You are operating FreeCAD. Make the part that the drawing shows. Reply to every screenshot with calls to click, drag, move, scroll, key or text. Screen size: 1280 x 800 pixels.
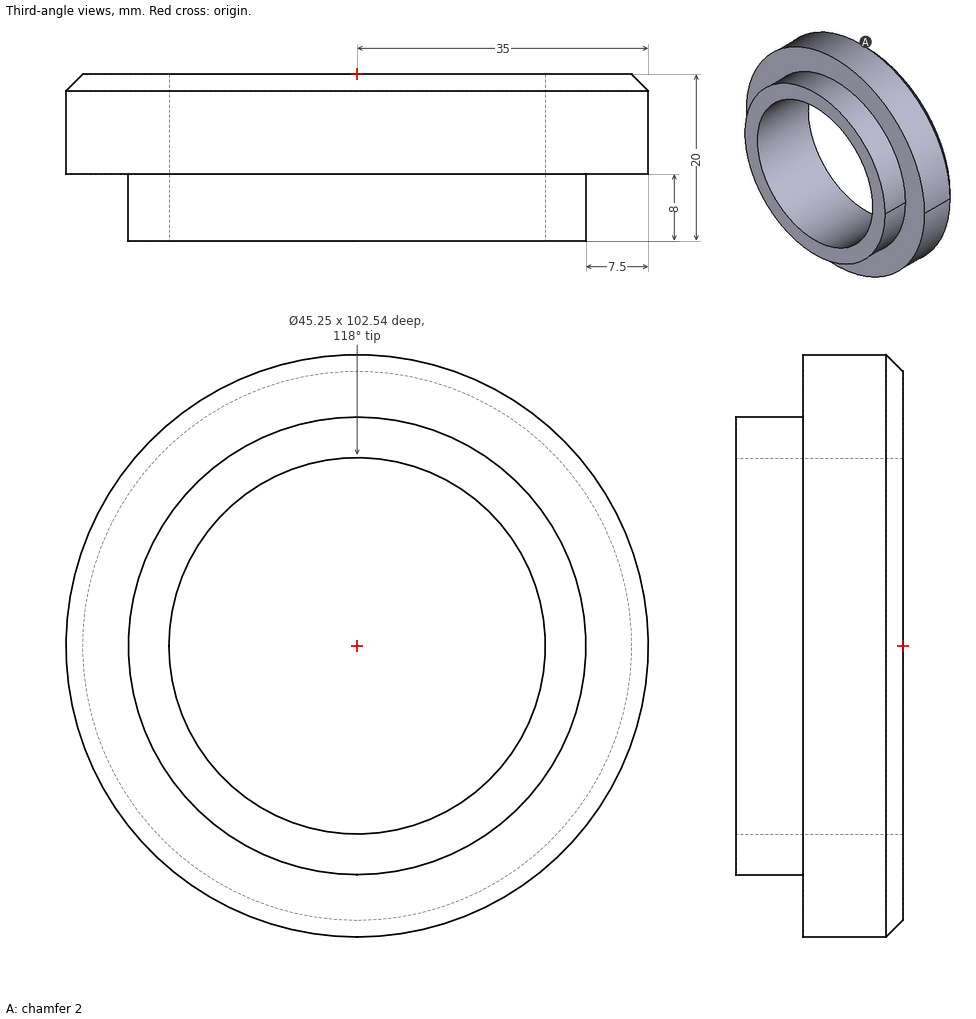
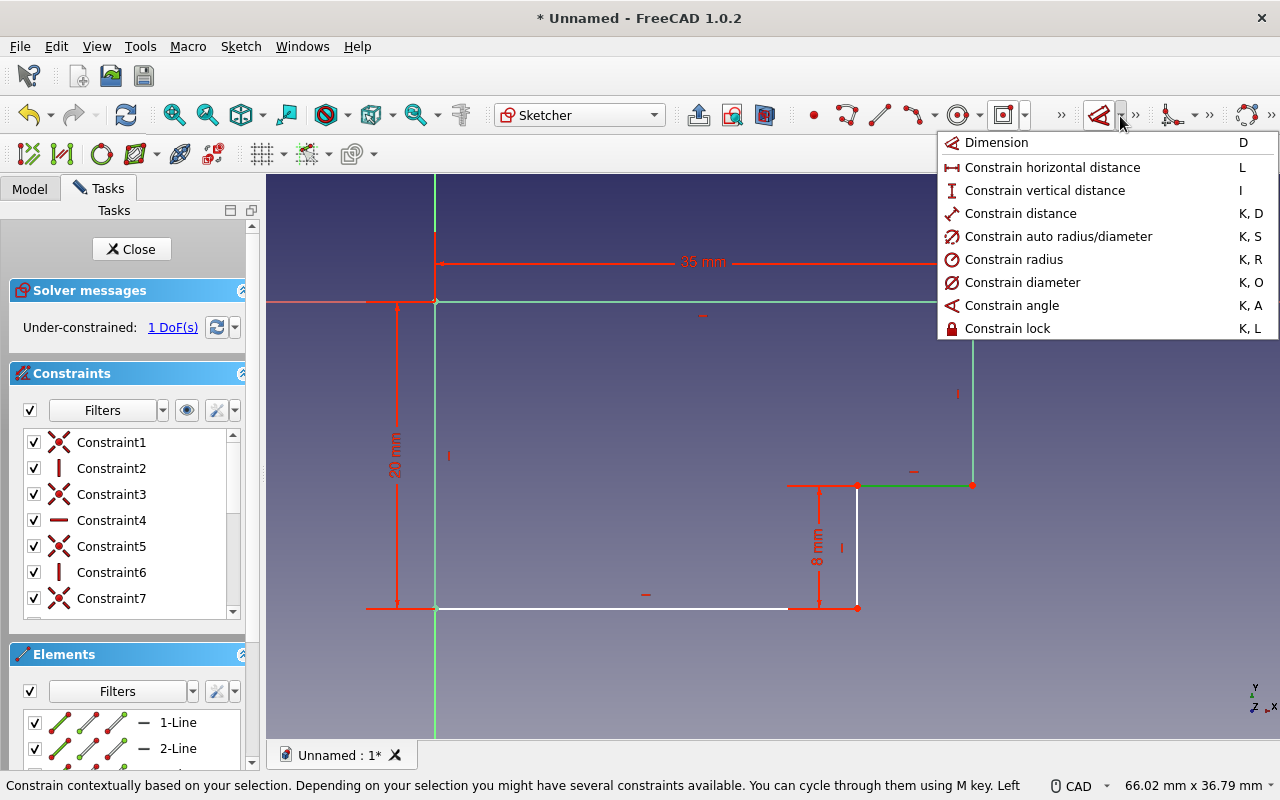
click(1108, 168)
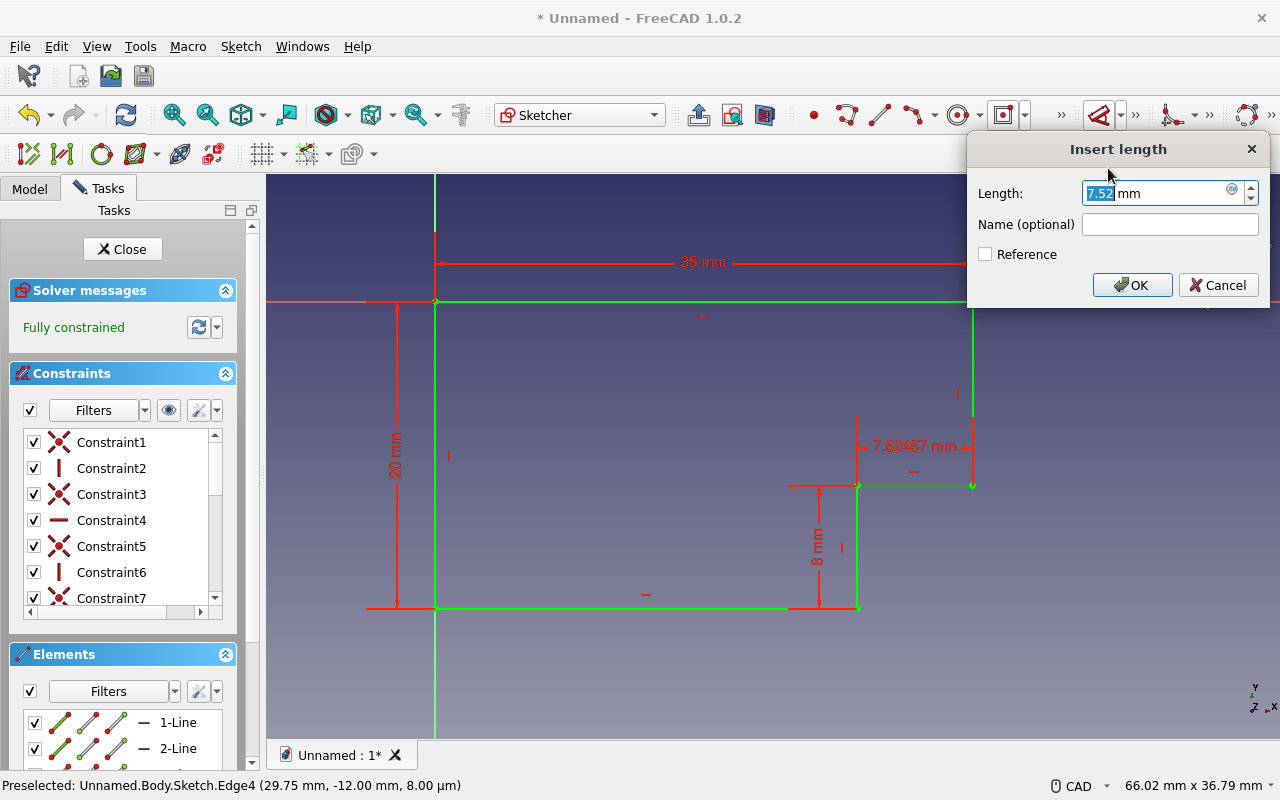
text(7.5)
key(Return)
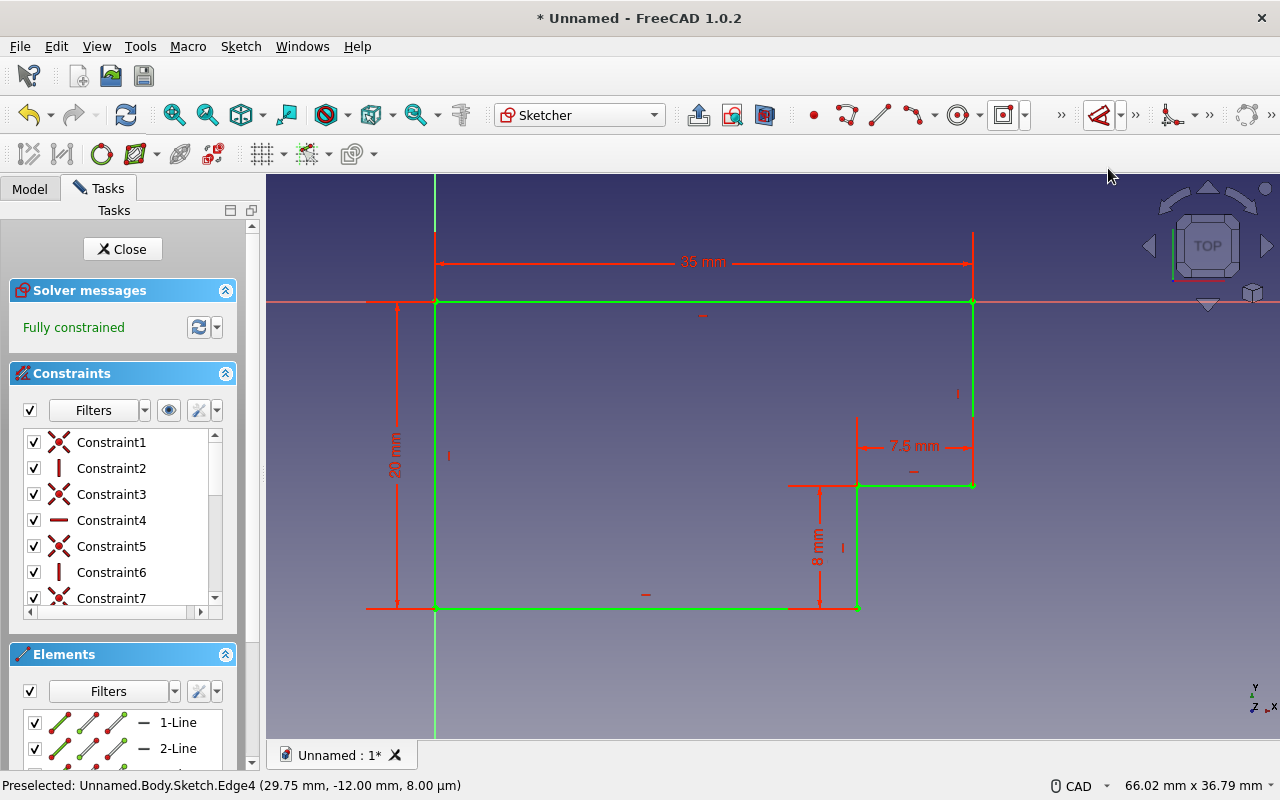
click(123, 249)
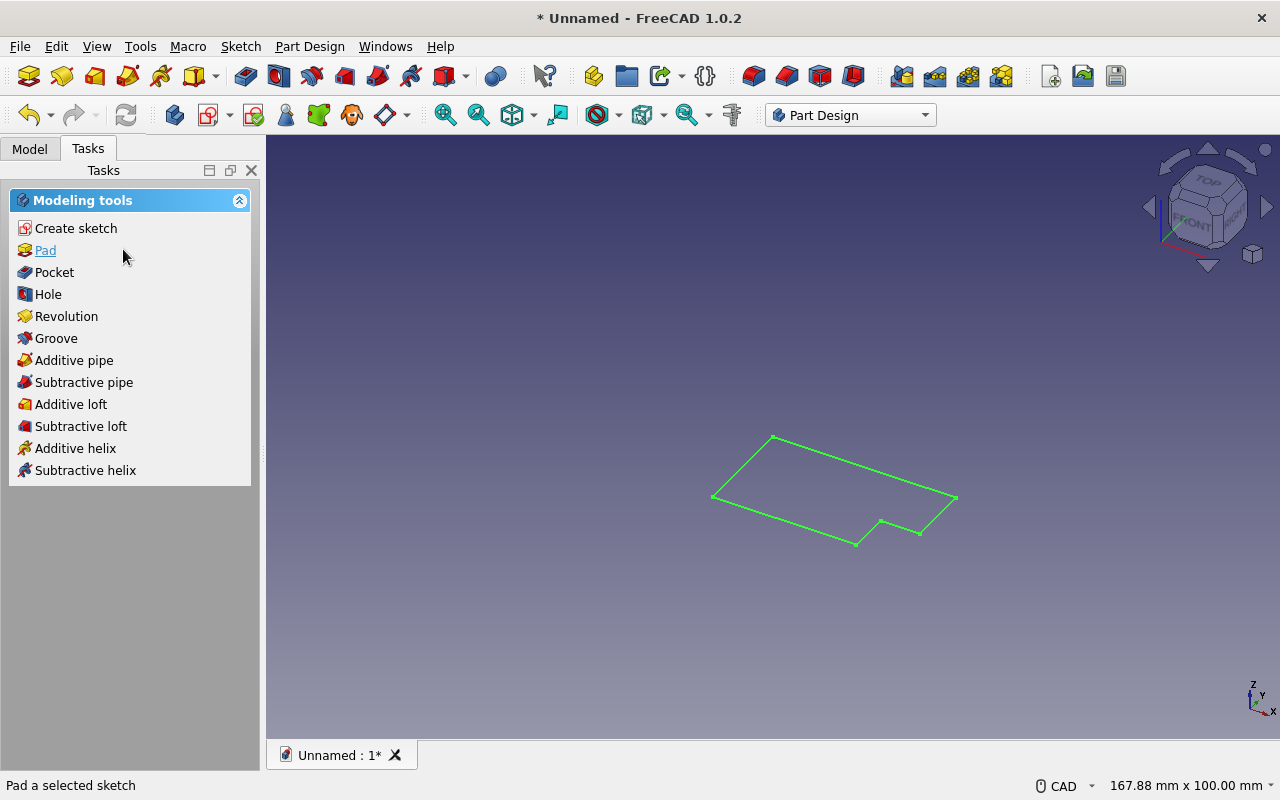
click(62, 76)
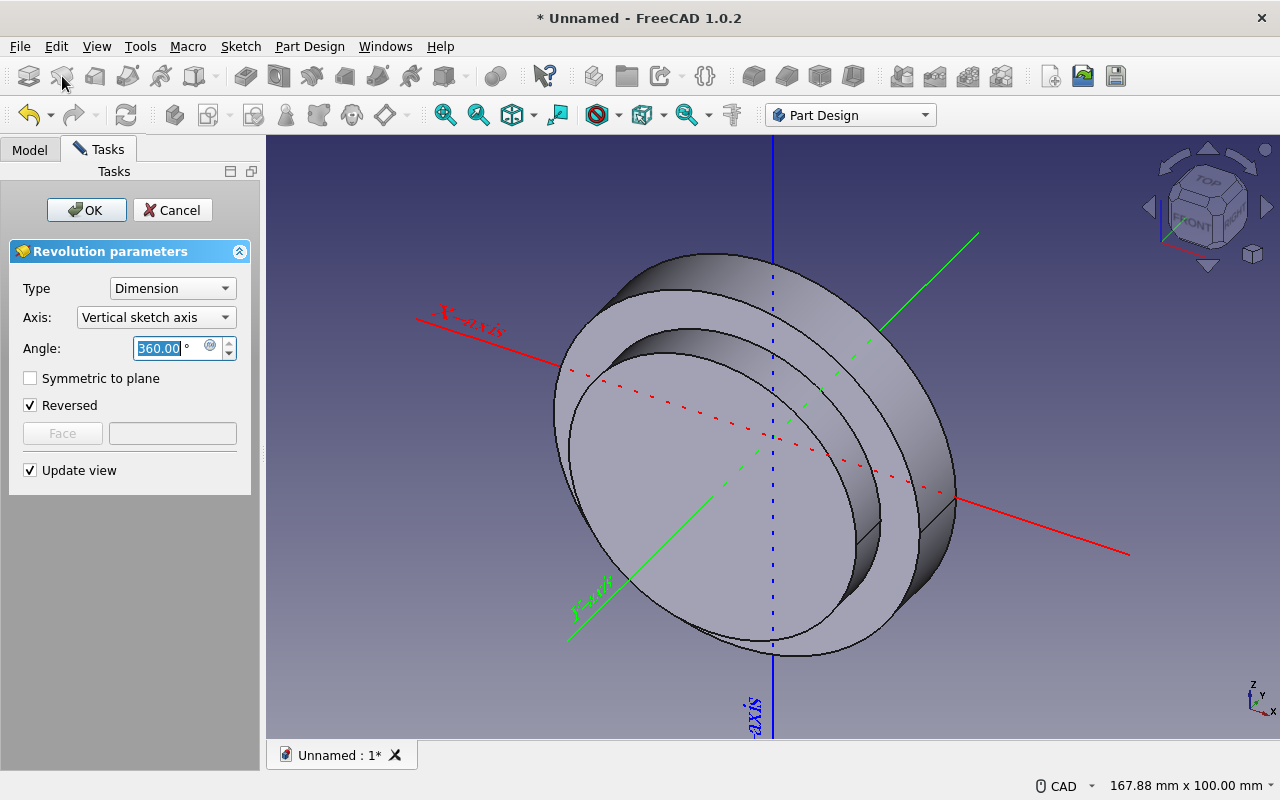
click(87, 210)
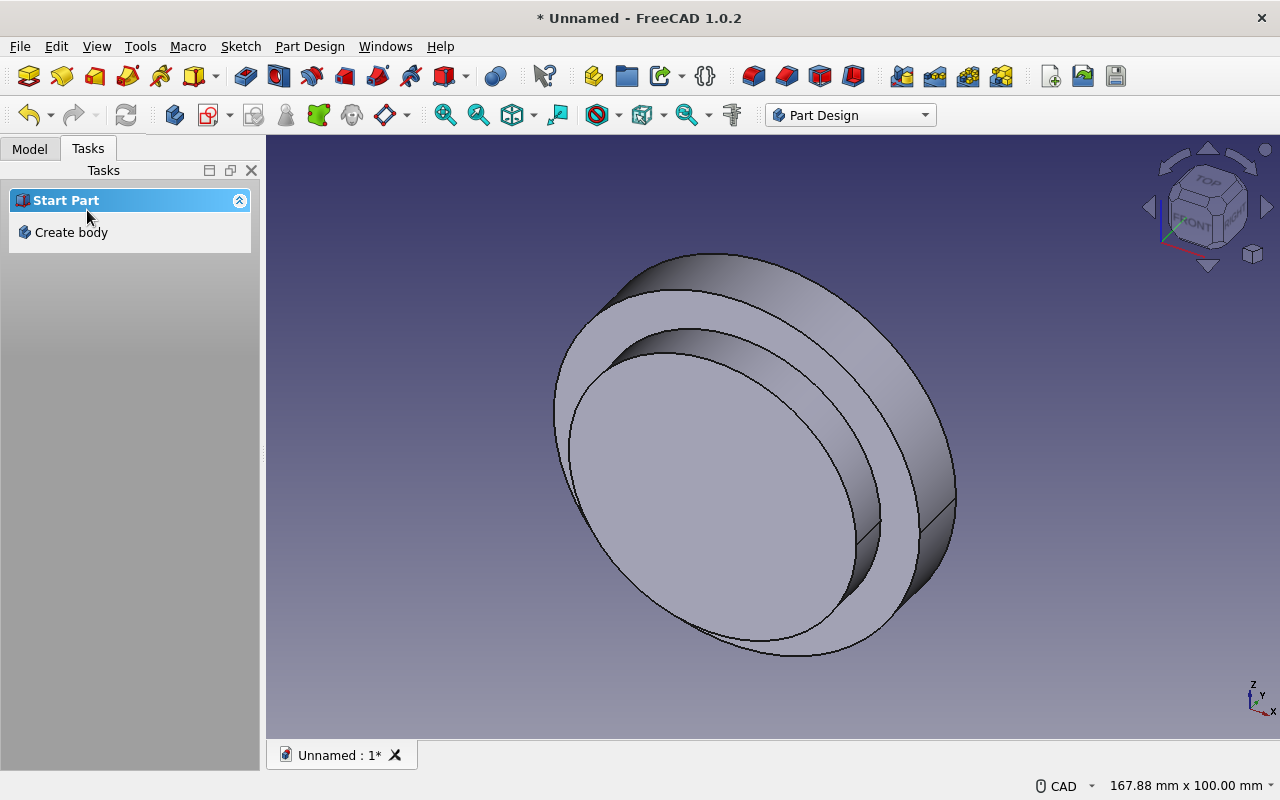
click(208, 116)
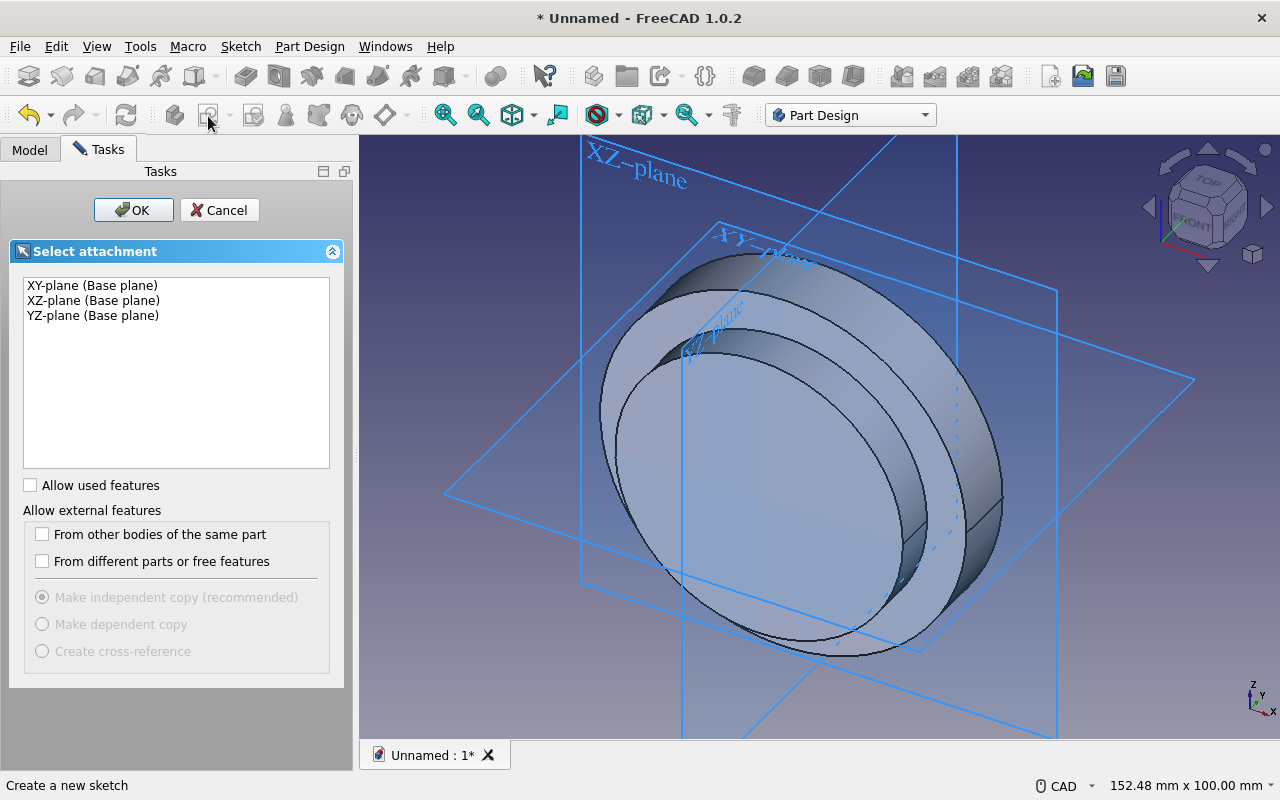
click(84, 300)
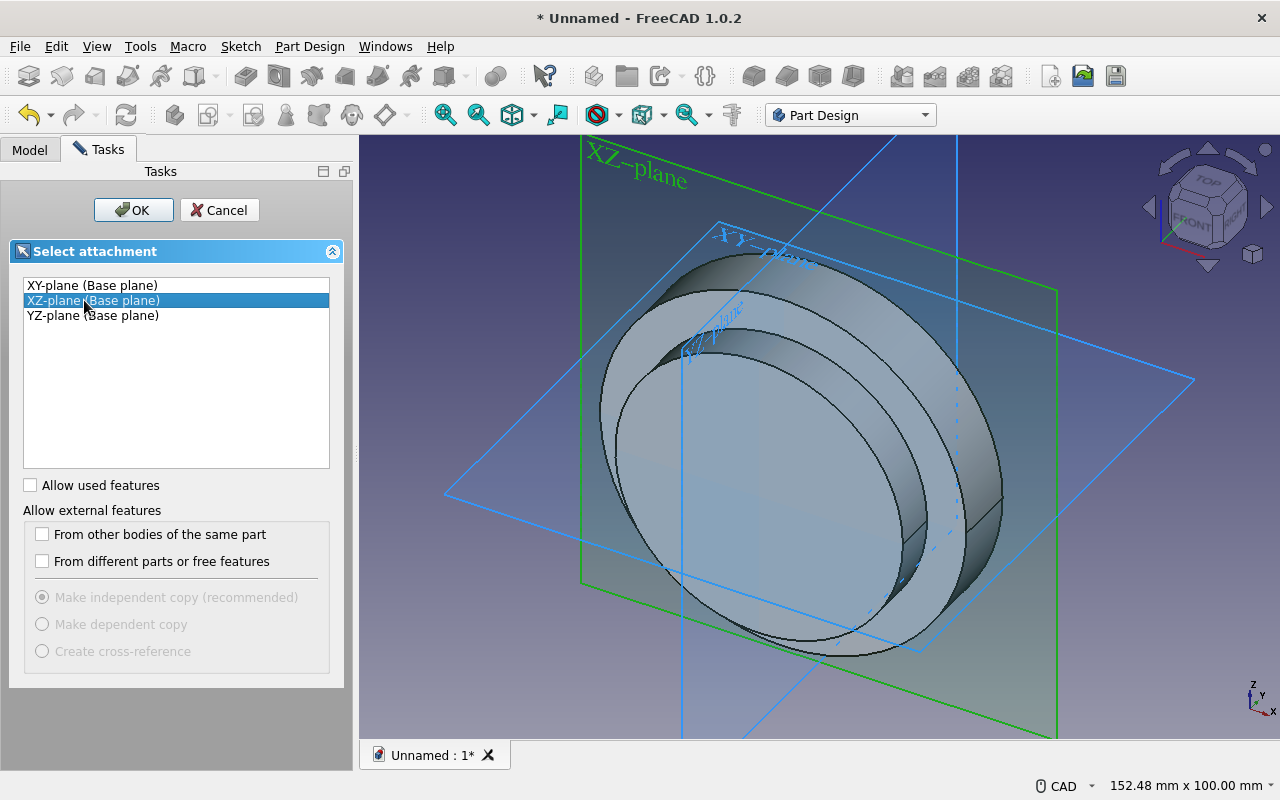
click(134, 210)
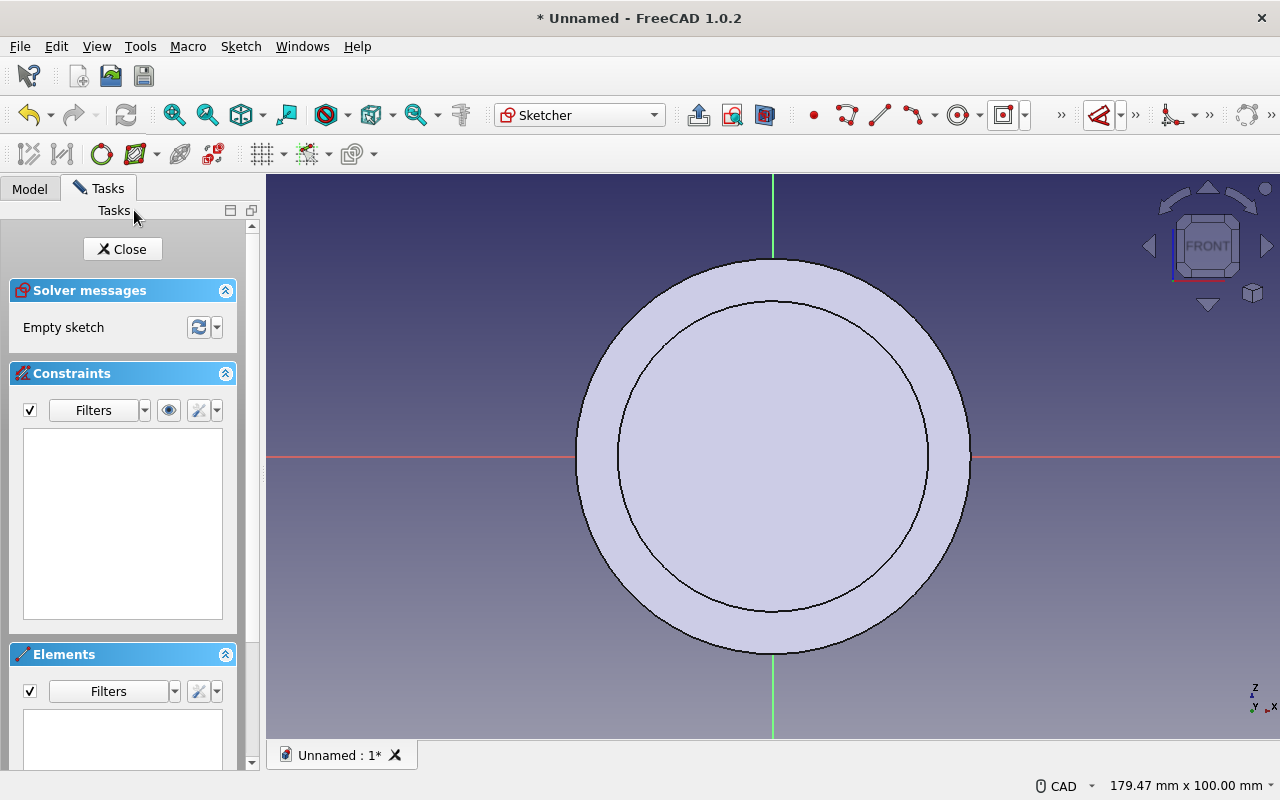
click(765, 116)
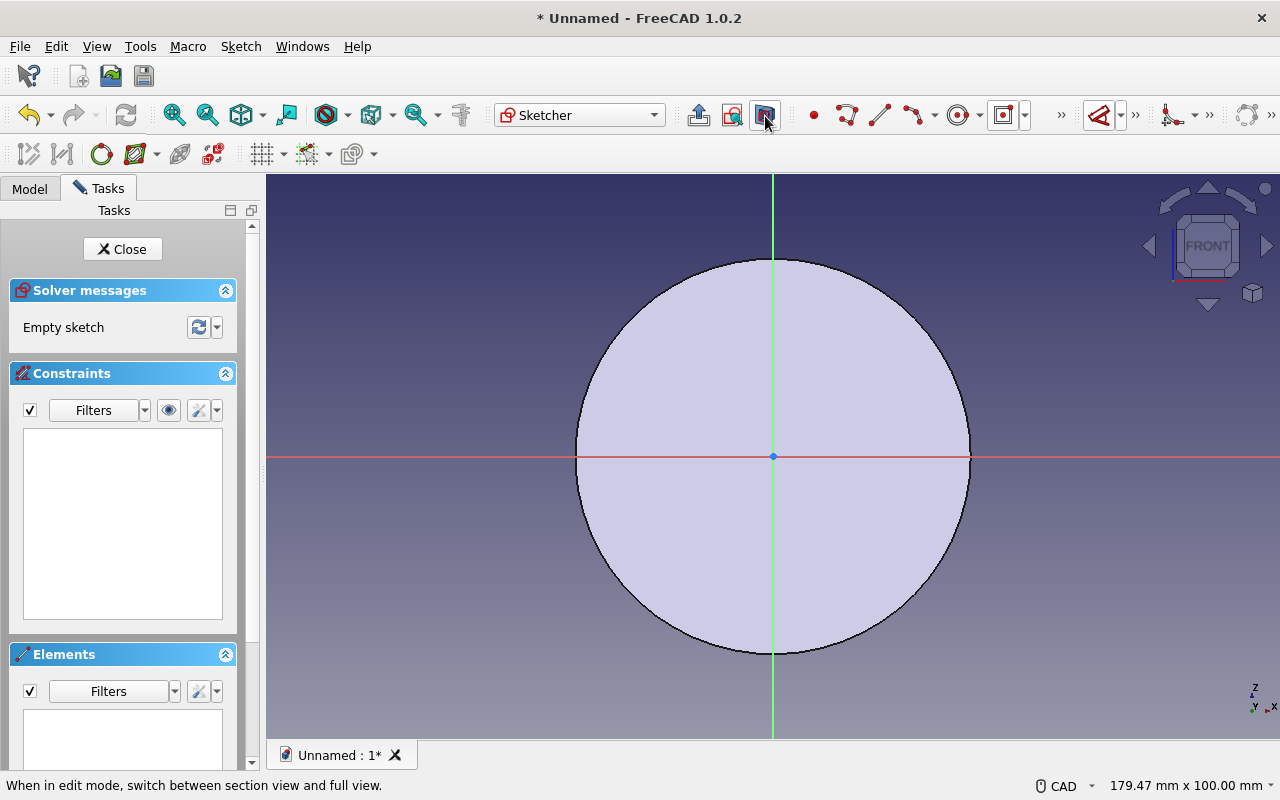
scroll(912, 456, up, 2)